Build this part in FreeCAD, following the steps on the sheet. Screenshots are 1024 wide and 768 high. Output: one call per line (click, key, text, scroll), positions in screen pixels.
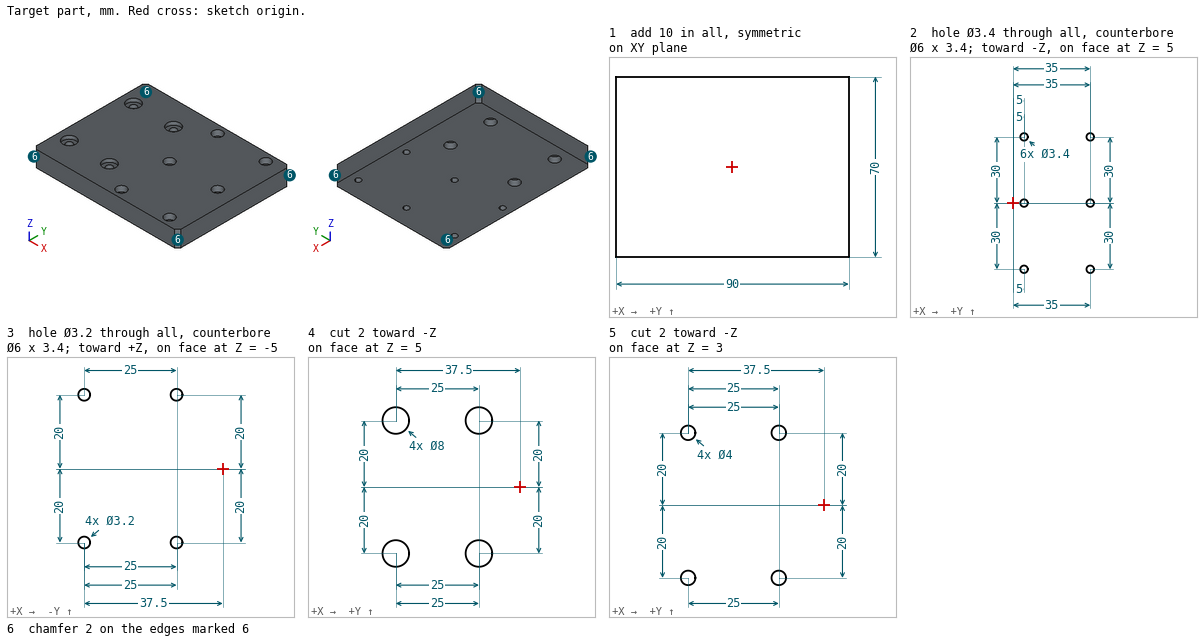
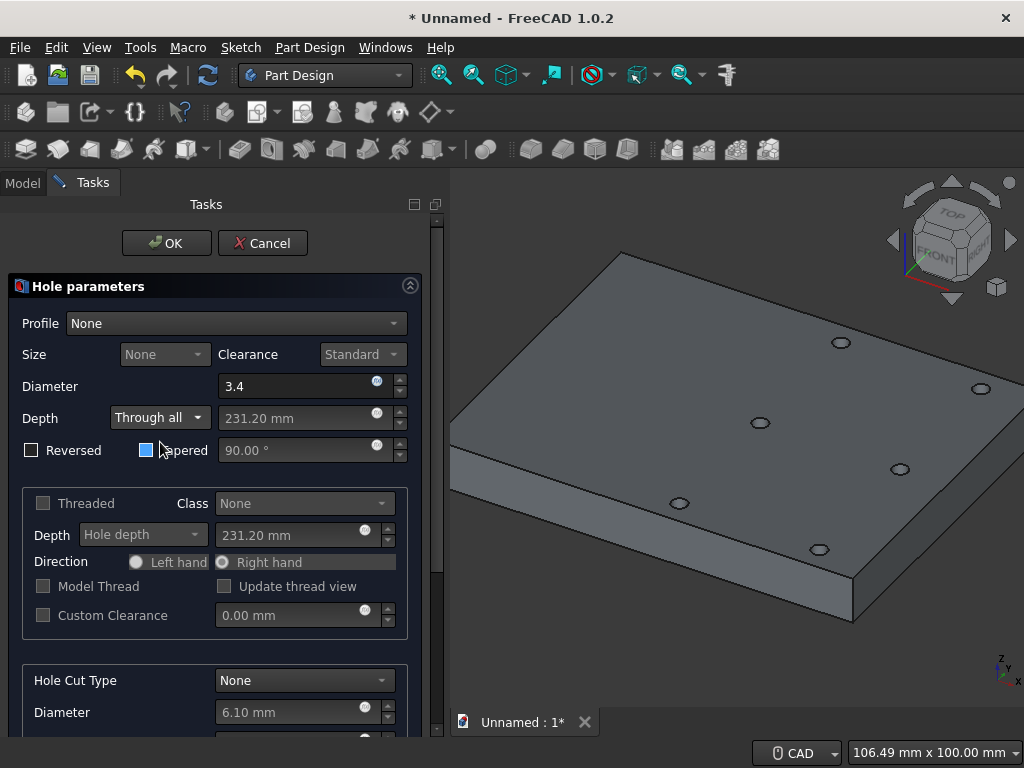
click(306, 680)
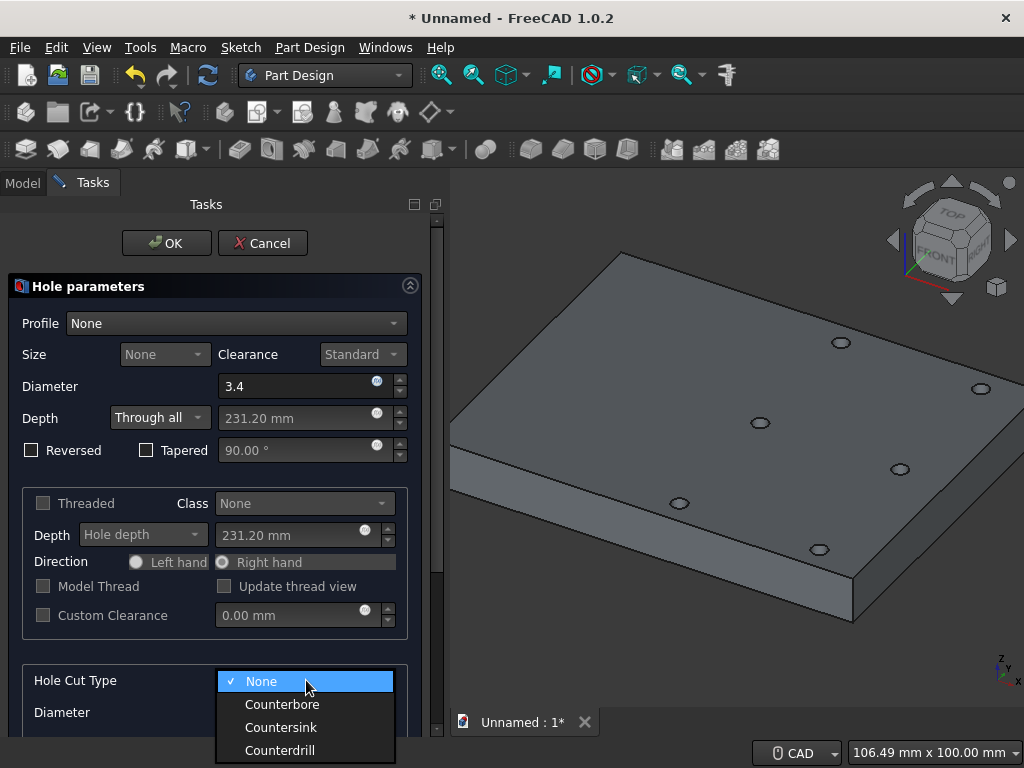
click(304, 704)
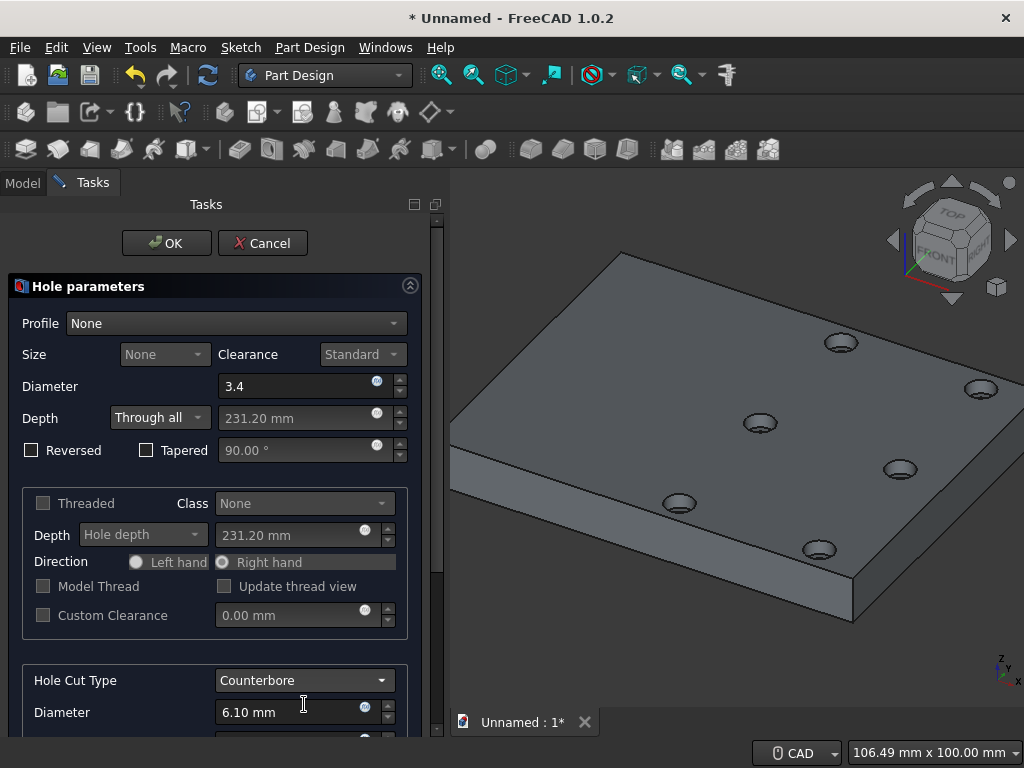
triple_click(298, 712)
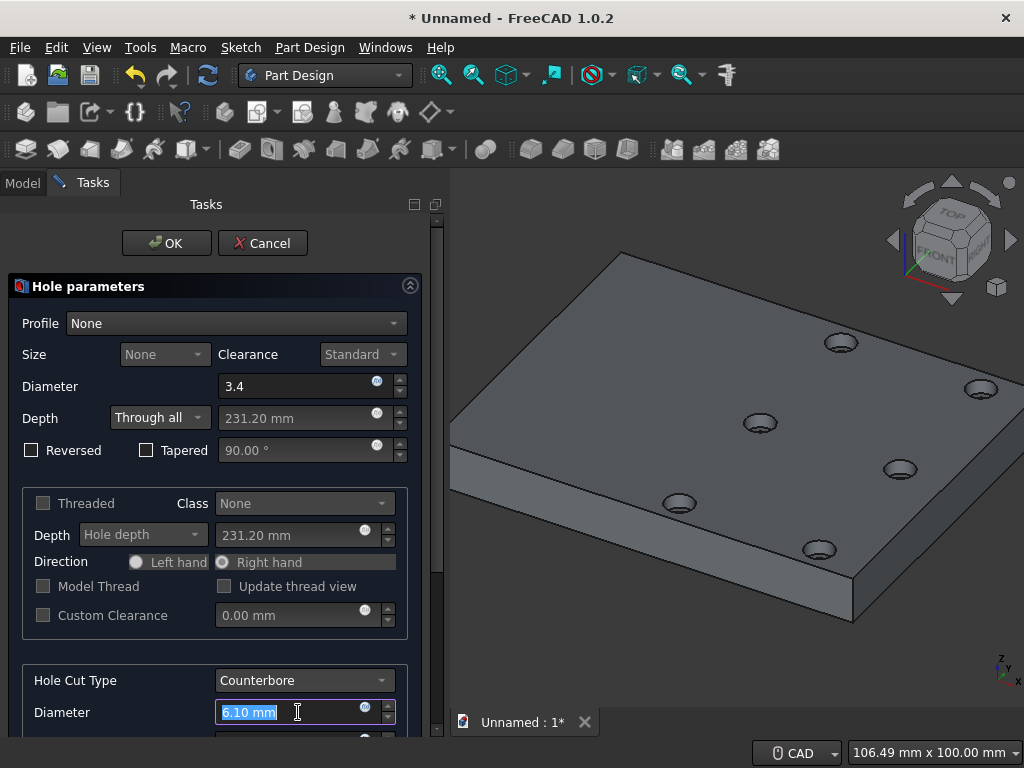
text(6)
key(Tab)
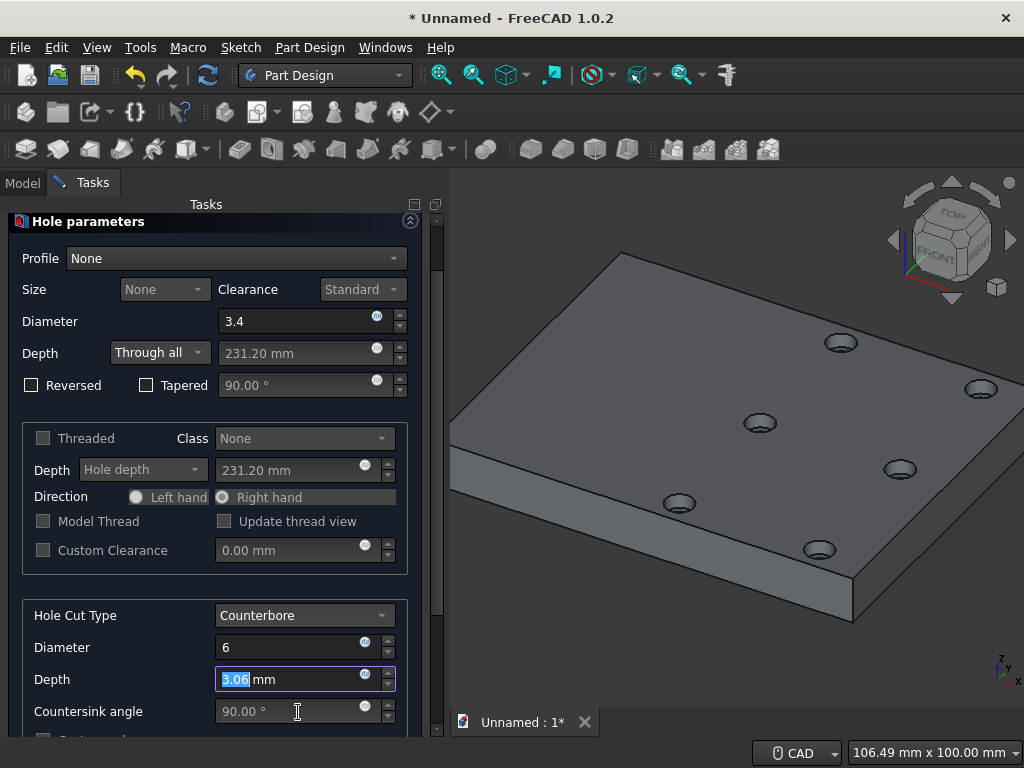
text(3.4)
key(Tab)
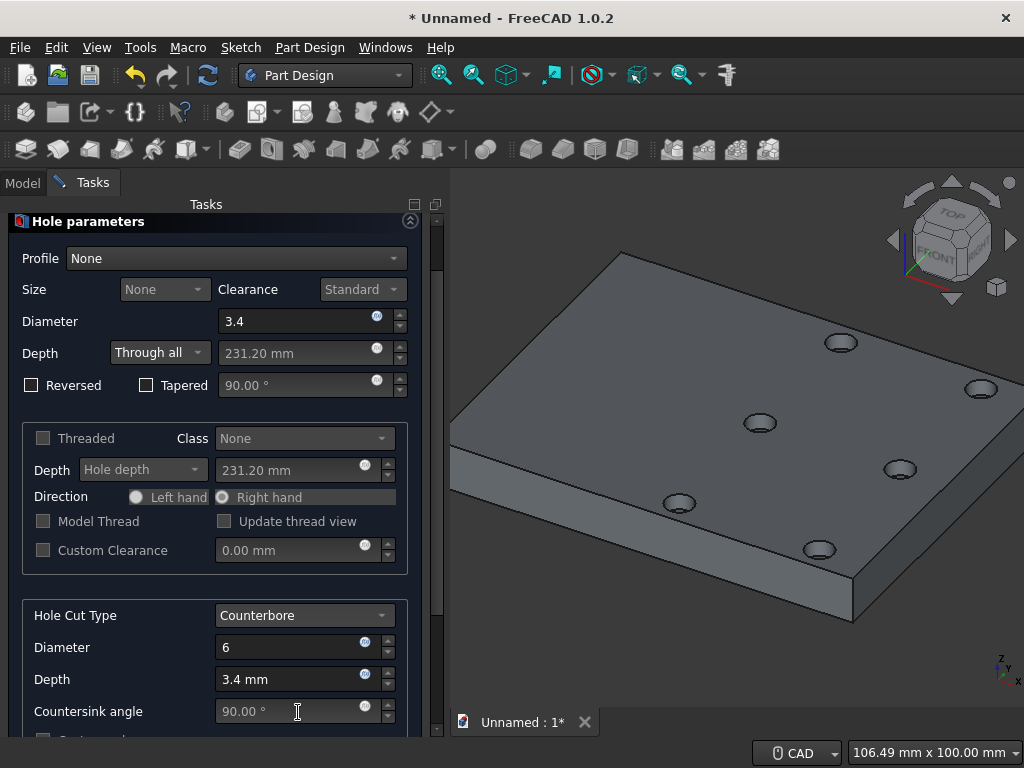
scroll(437, 475, up, 2)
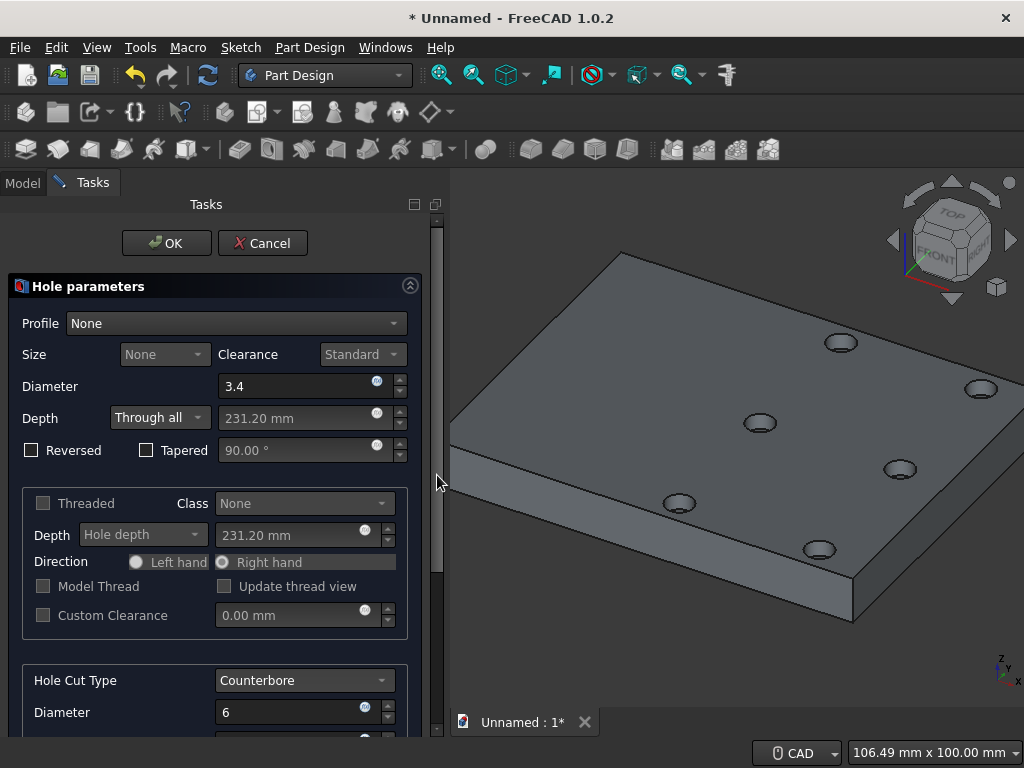
click(167, 243)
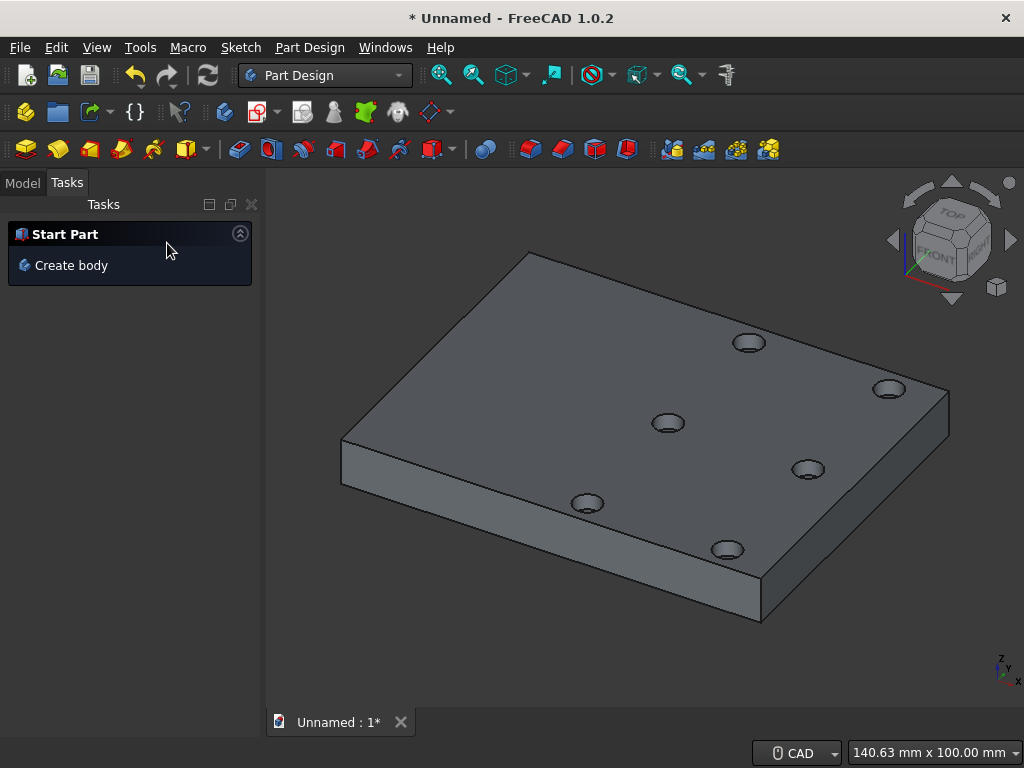
key(5)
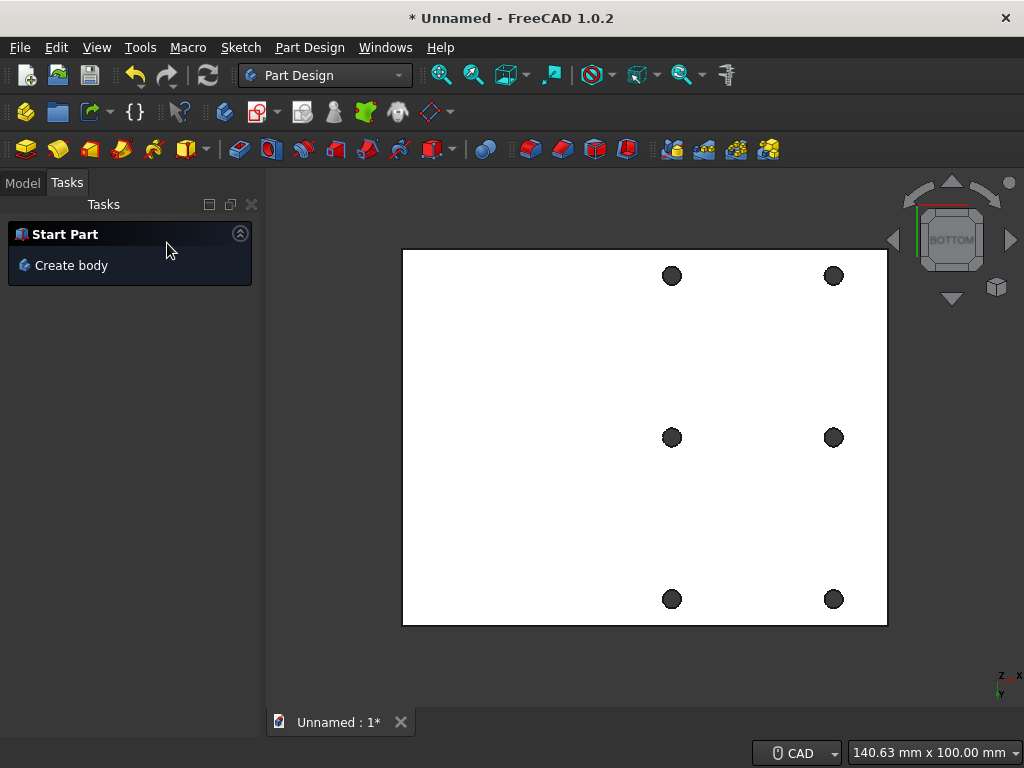
click(506, 490)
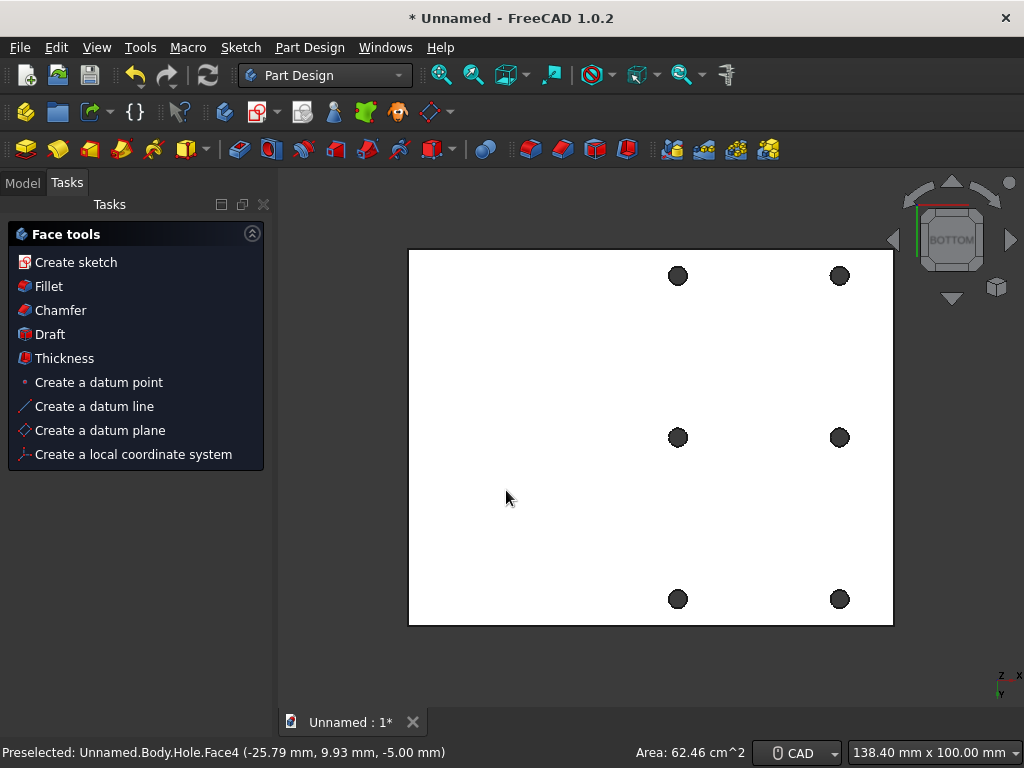
click(258, 112)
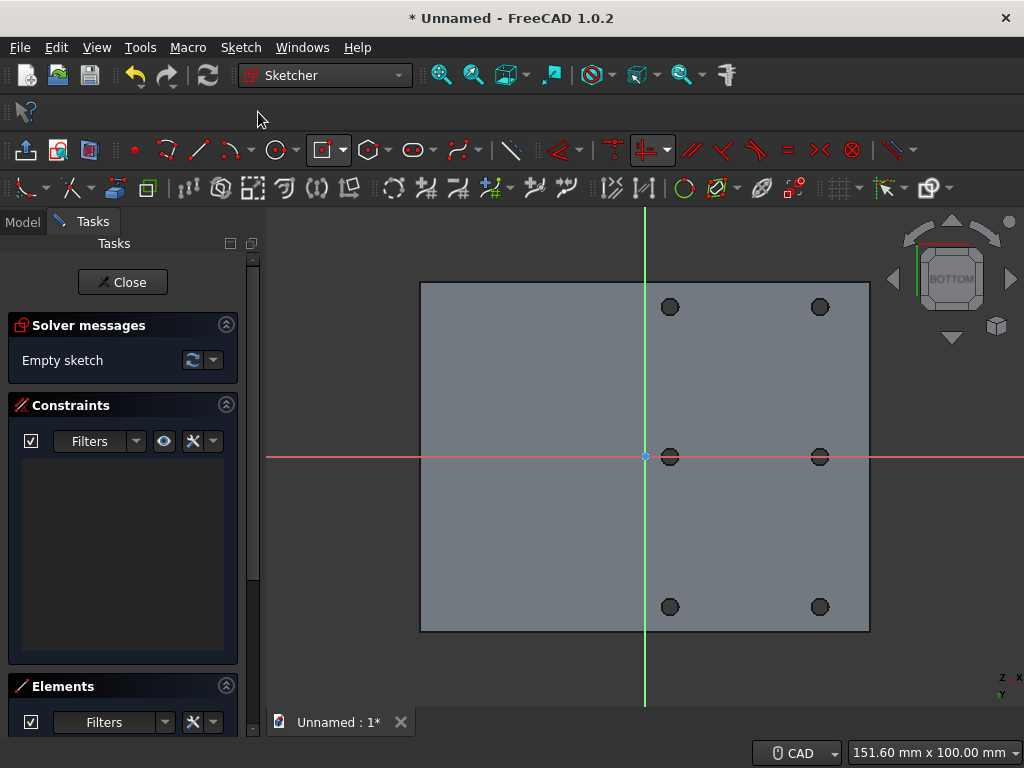
scroll(488, 457, up, 2)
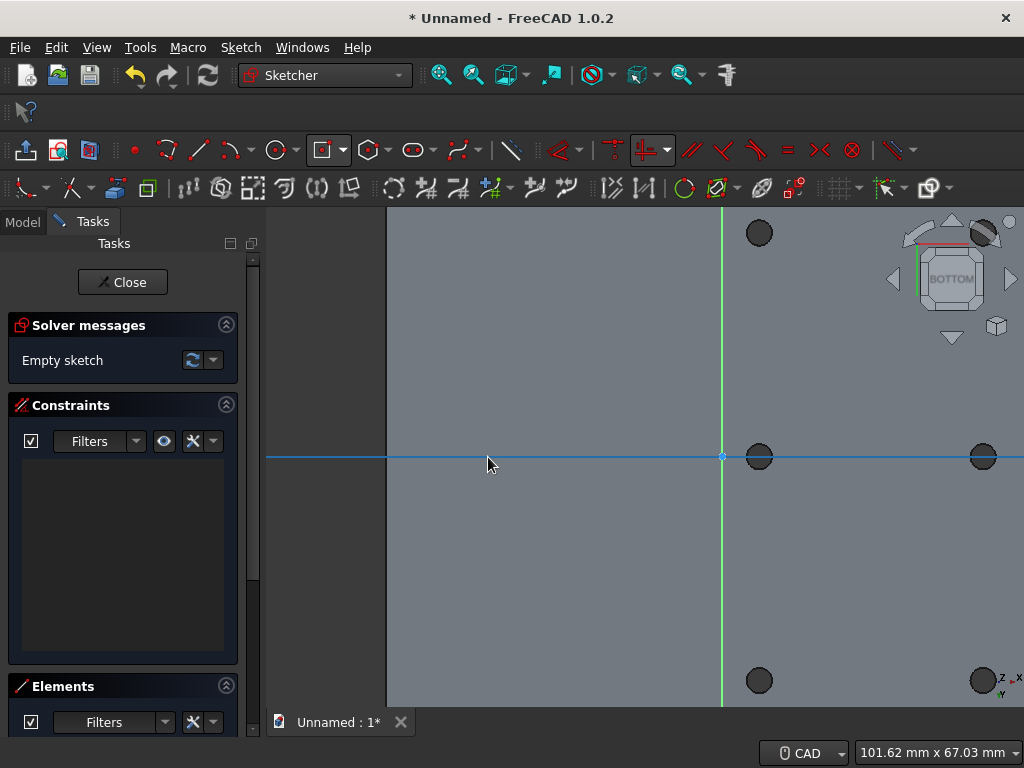
click(276, 150)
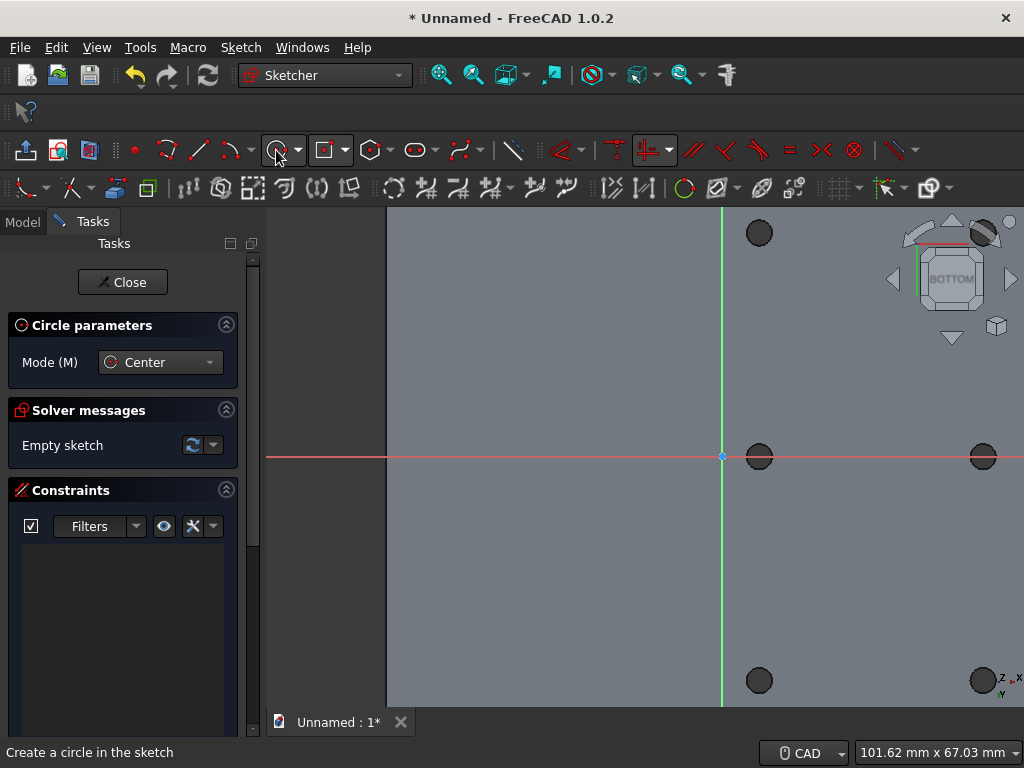
scroll(442, 606, up, 4)